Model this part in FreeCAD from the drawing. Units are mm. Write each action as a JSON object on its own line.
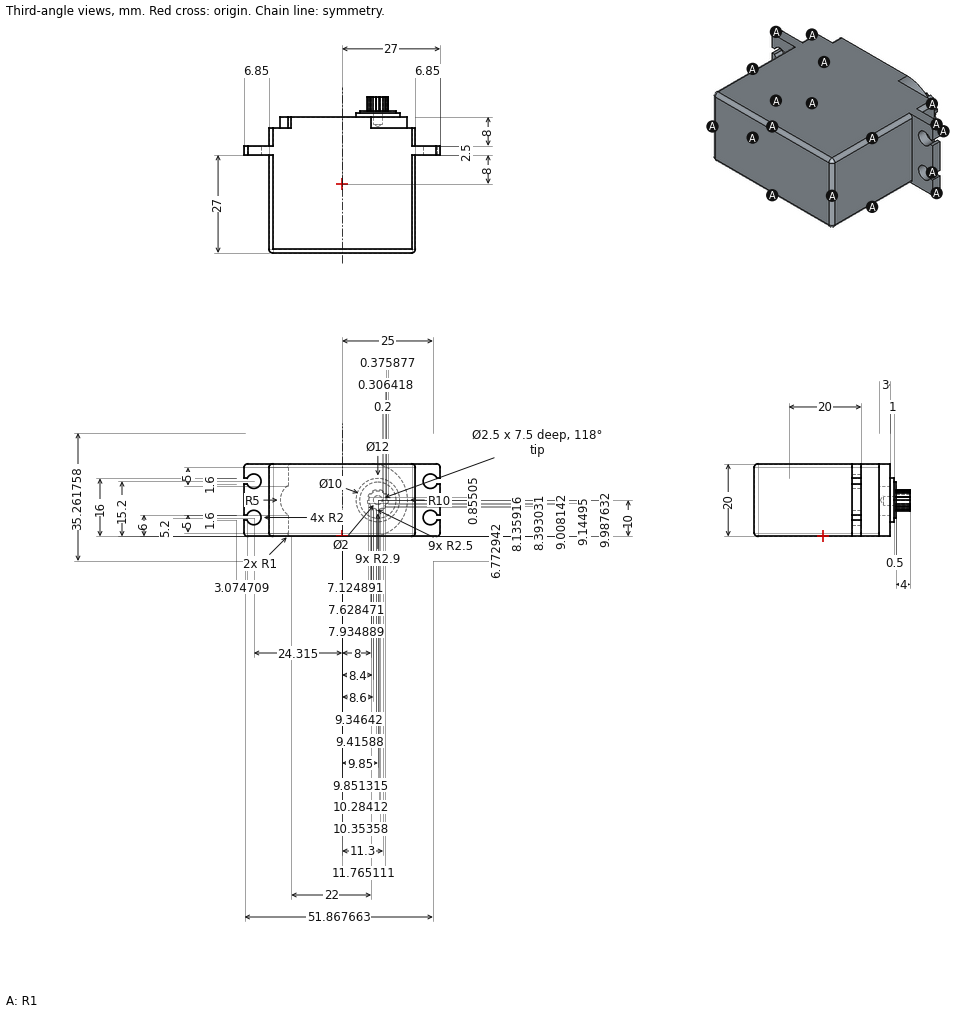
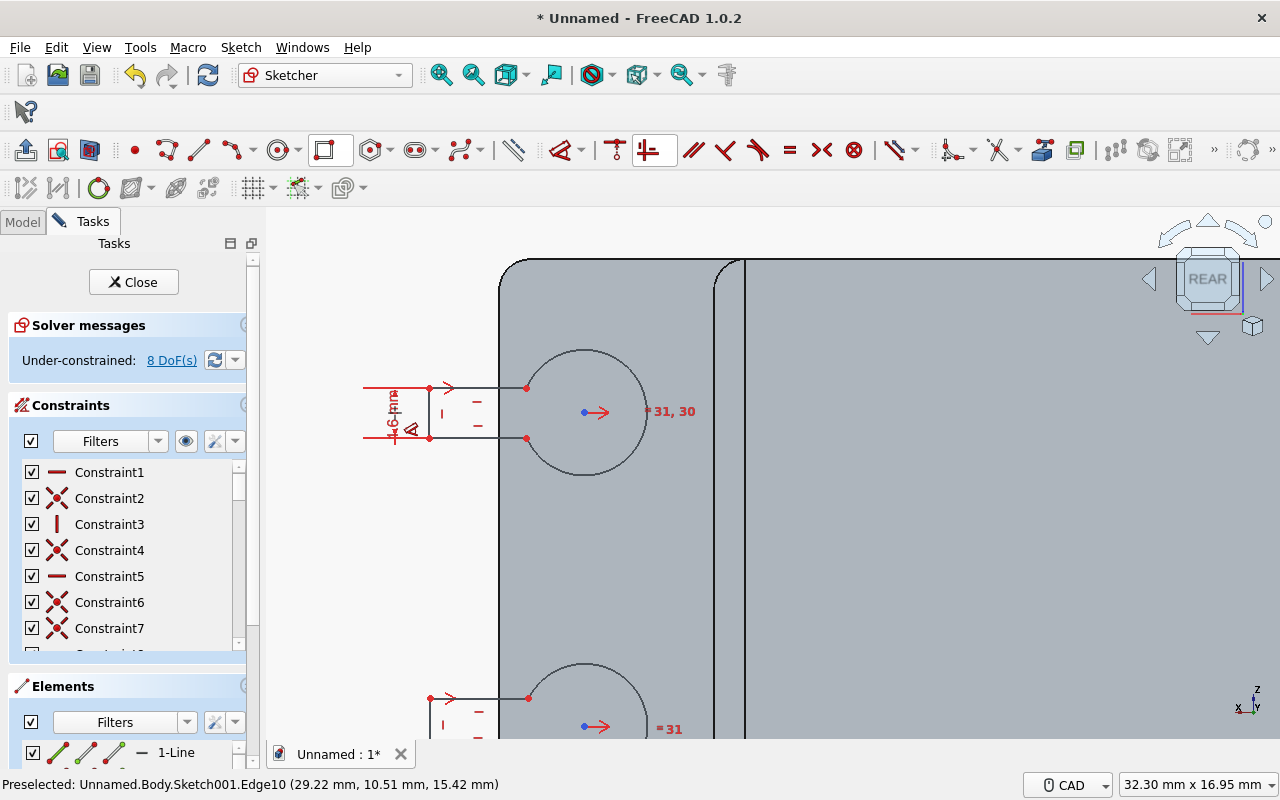
{"action": "scroll", "coordinate": [430, 709], "scroll_direction": "up", "scroll_amount": 2}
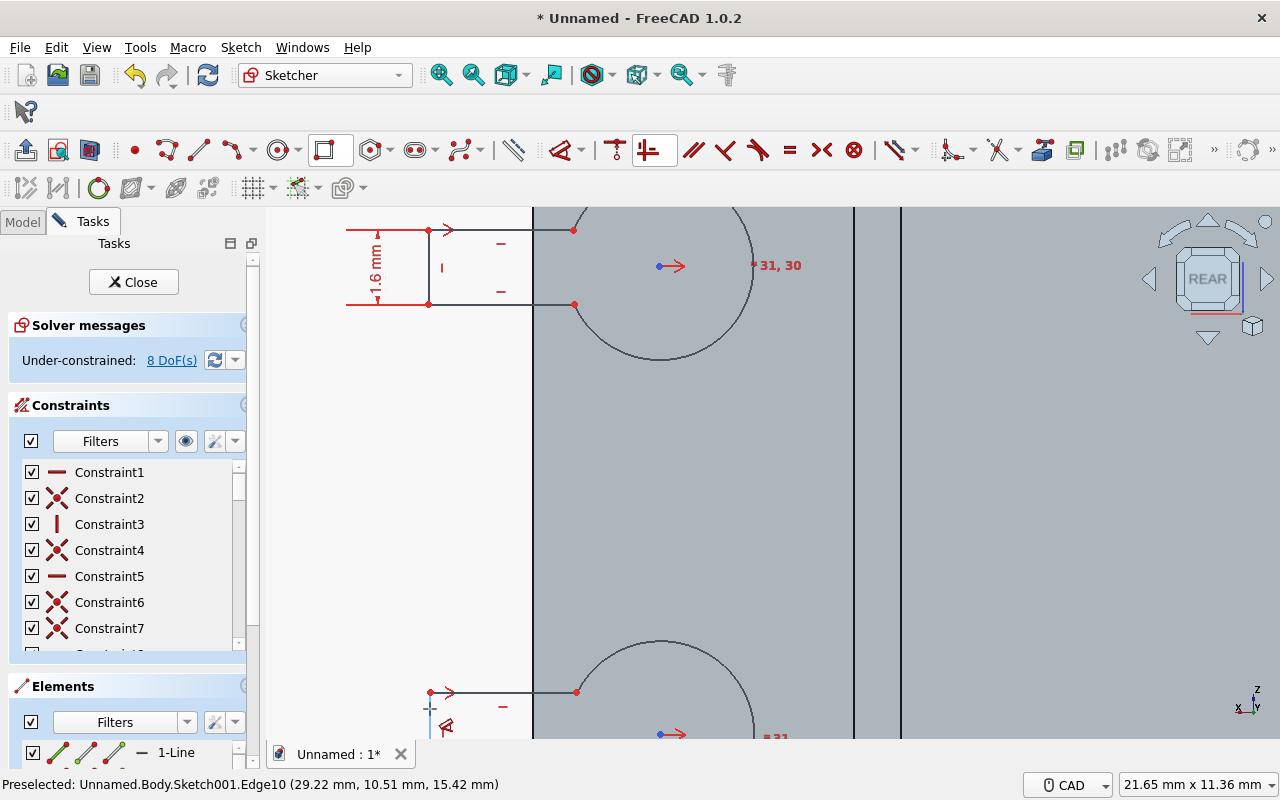
{"action": "left_click", "coordinate": [430, 709]}
{"action": "left_click", "coordinate": [396, 702]}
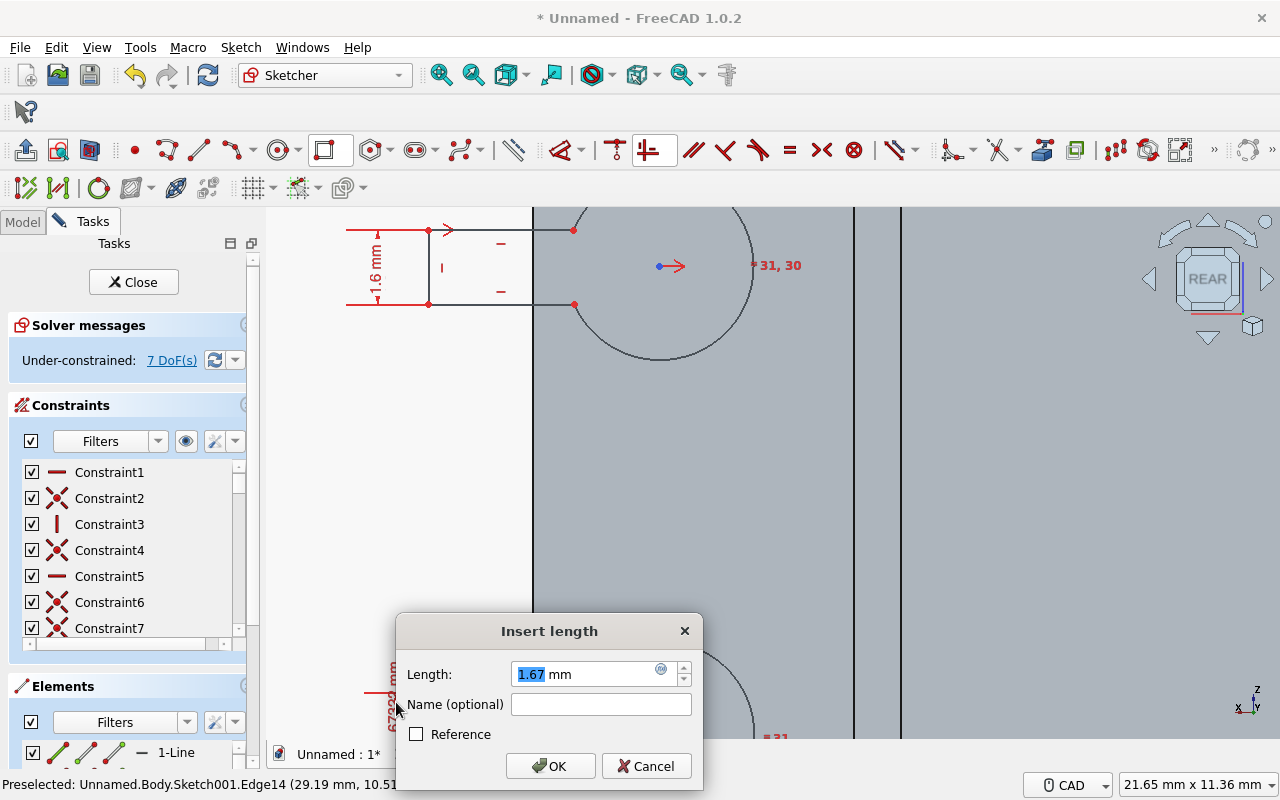
{"action": "type", "text": "1.6"}
{"action": "key", "text": "Return"}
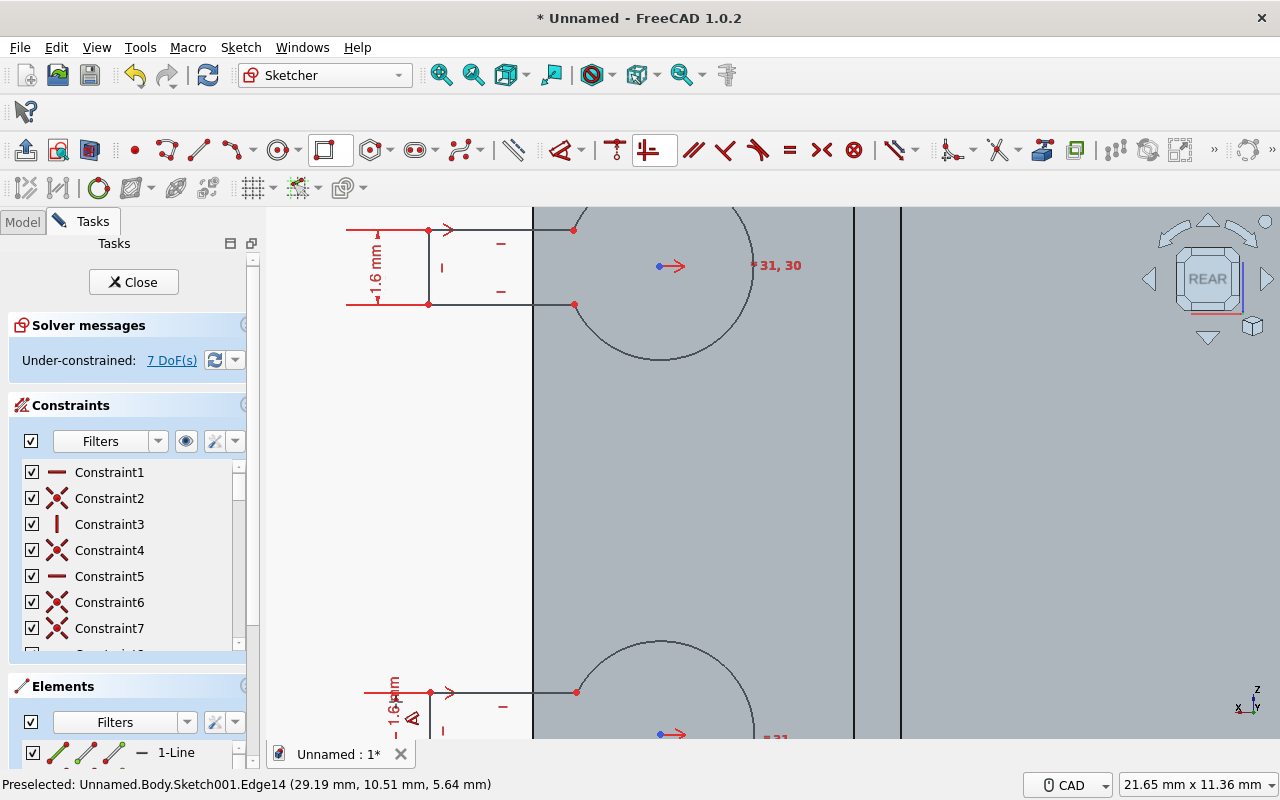
{"action": "scroll", "coordinate": [428, 441], "scroll_direction": "down", "scroll_amount": 8}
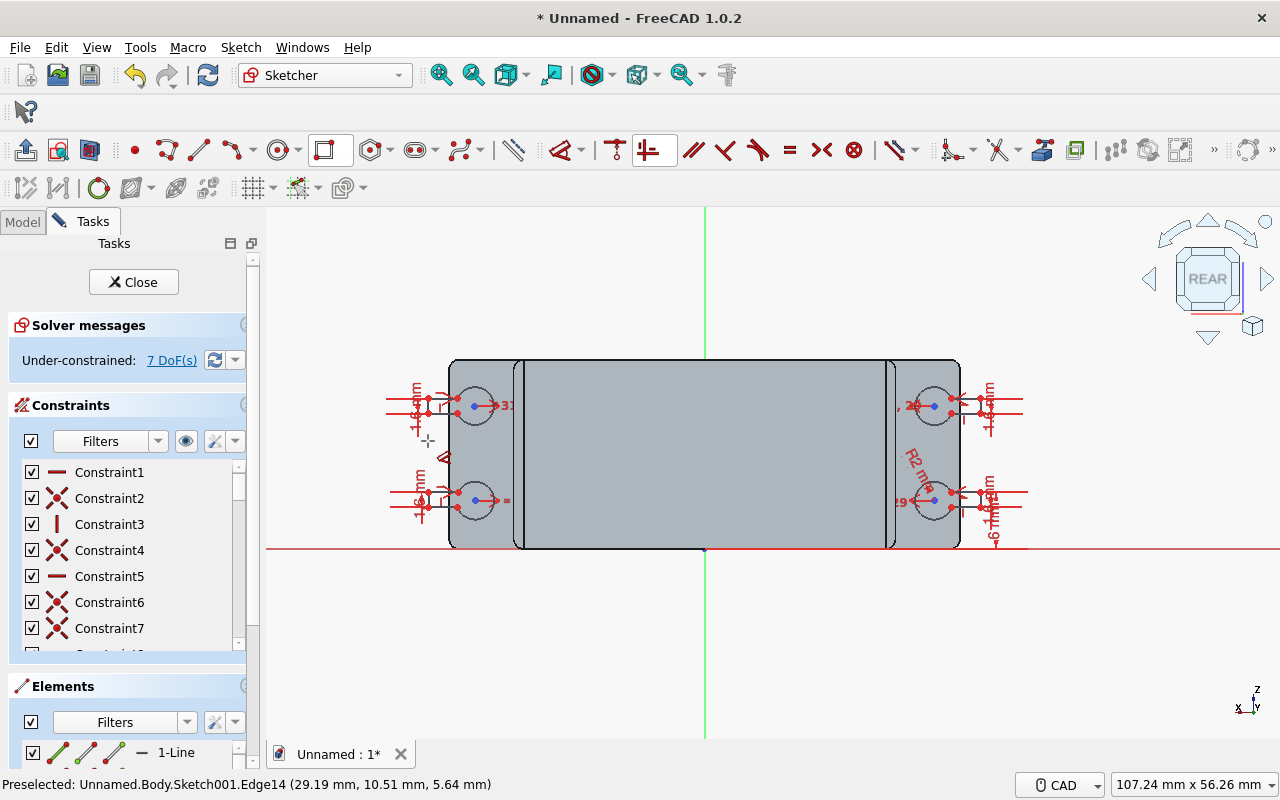
{"action": "left_click", "coordinate": [981, 399]}
{"action": "left_click", "coordinate": [1015, 474]}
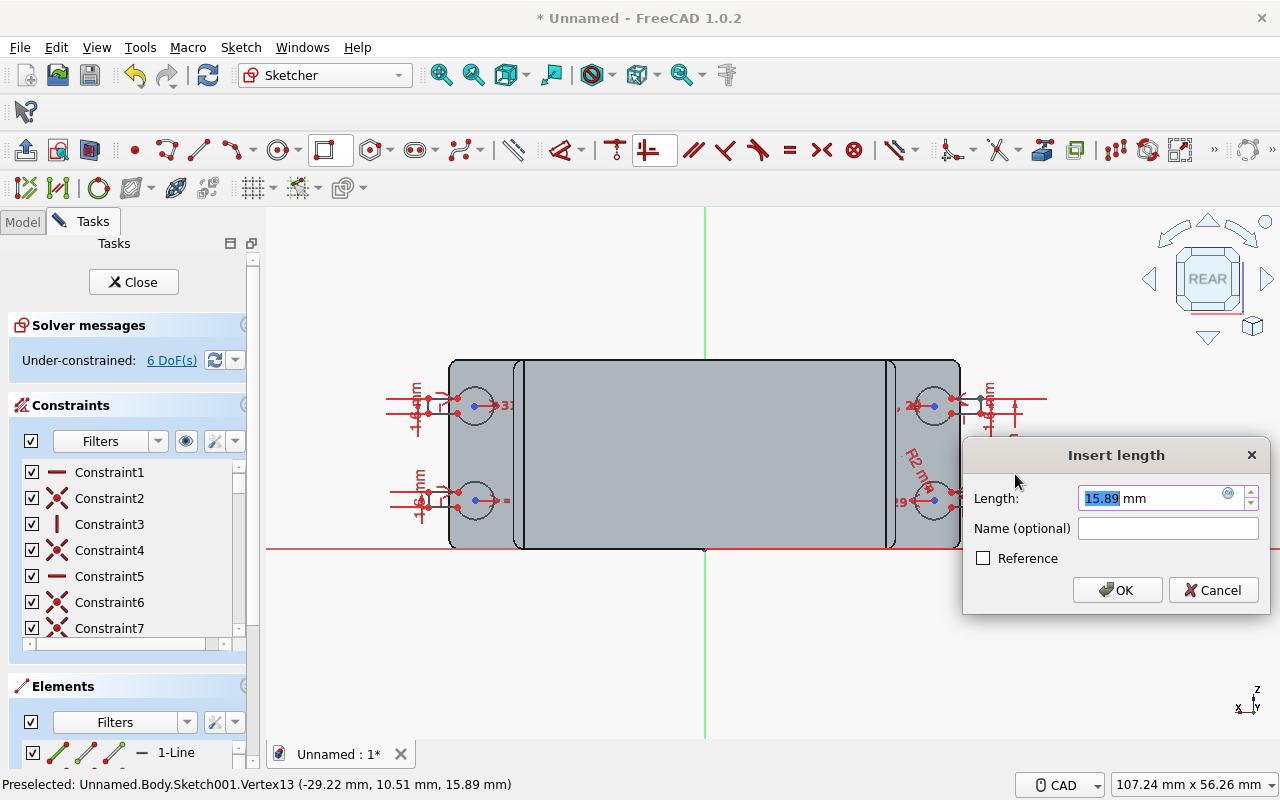
{"action": "type", "text": "16"}
{"action": "key", "text": "Return"}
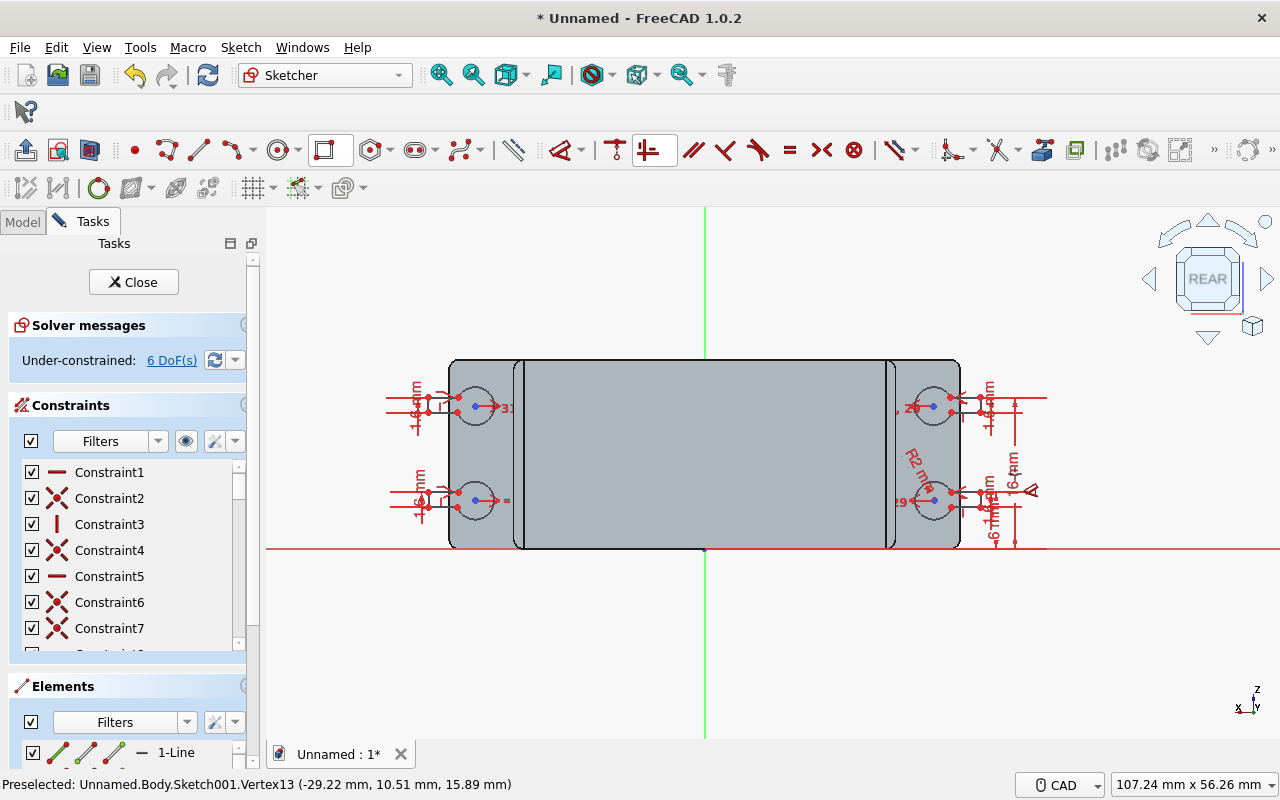
{"action": "left_click", "coordinate": [934, 501]}
{"action": "left_click", "coordinate": [671, 525]}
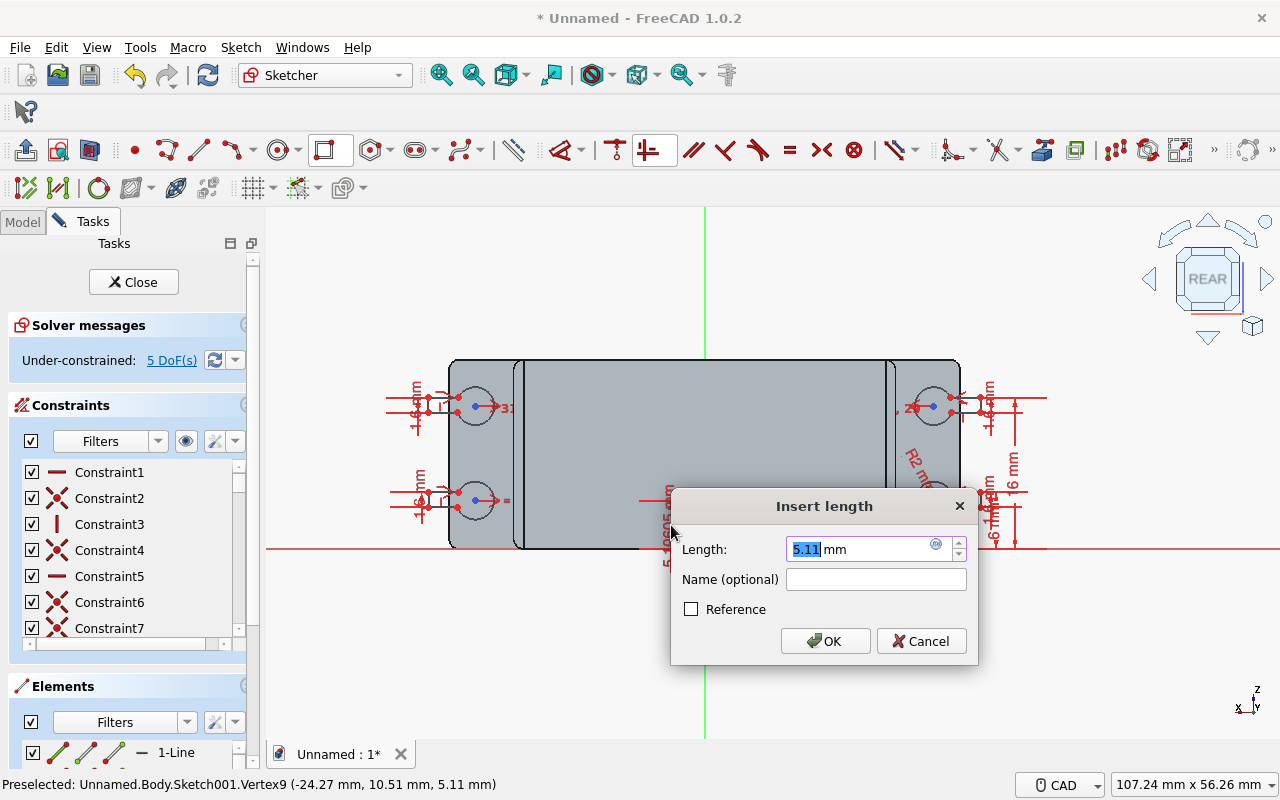
{"action": "type", "text": "5.2"}
{"action": "key", "text": "Return"}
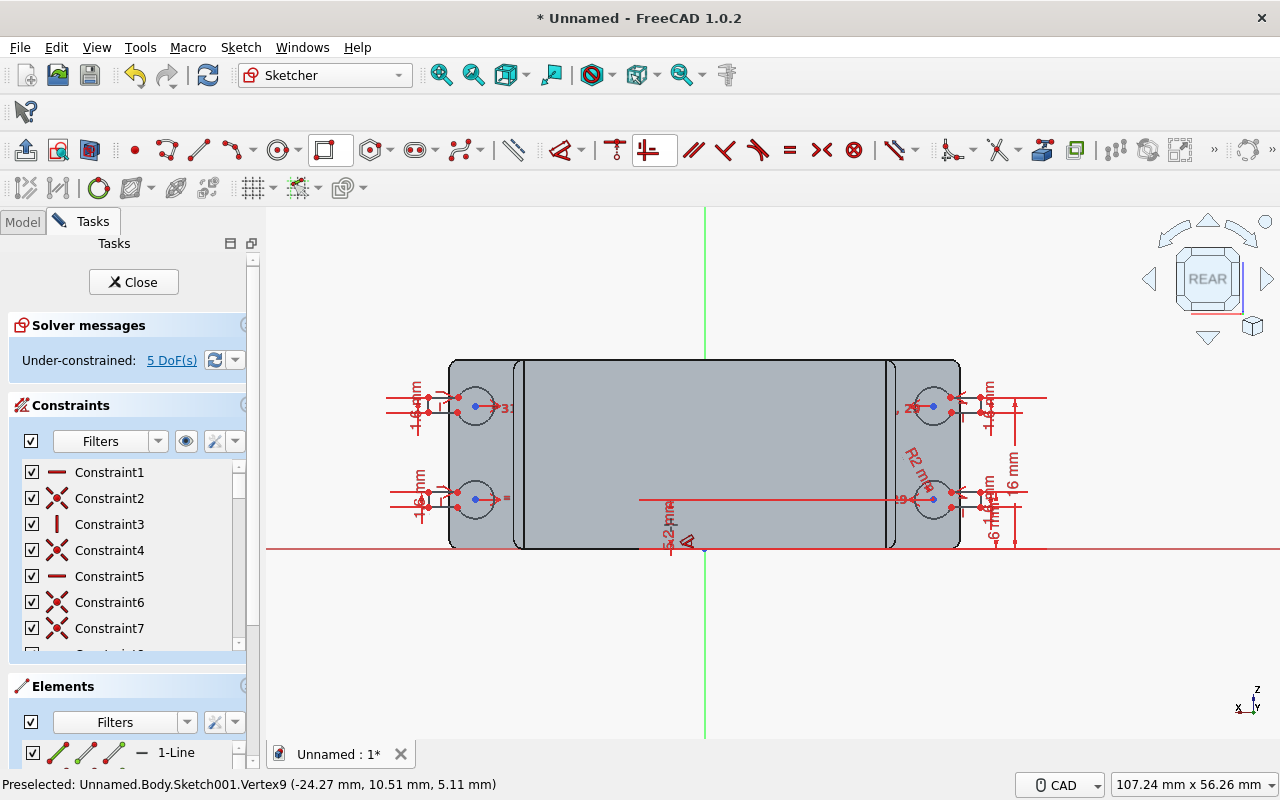
{"action": "left_click", "coordinate": [934, 406]}
{"action": "left_click", "coordinate": [968, 445]}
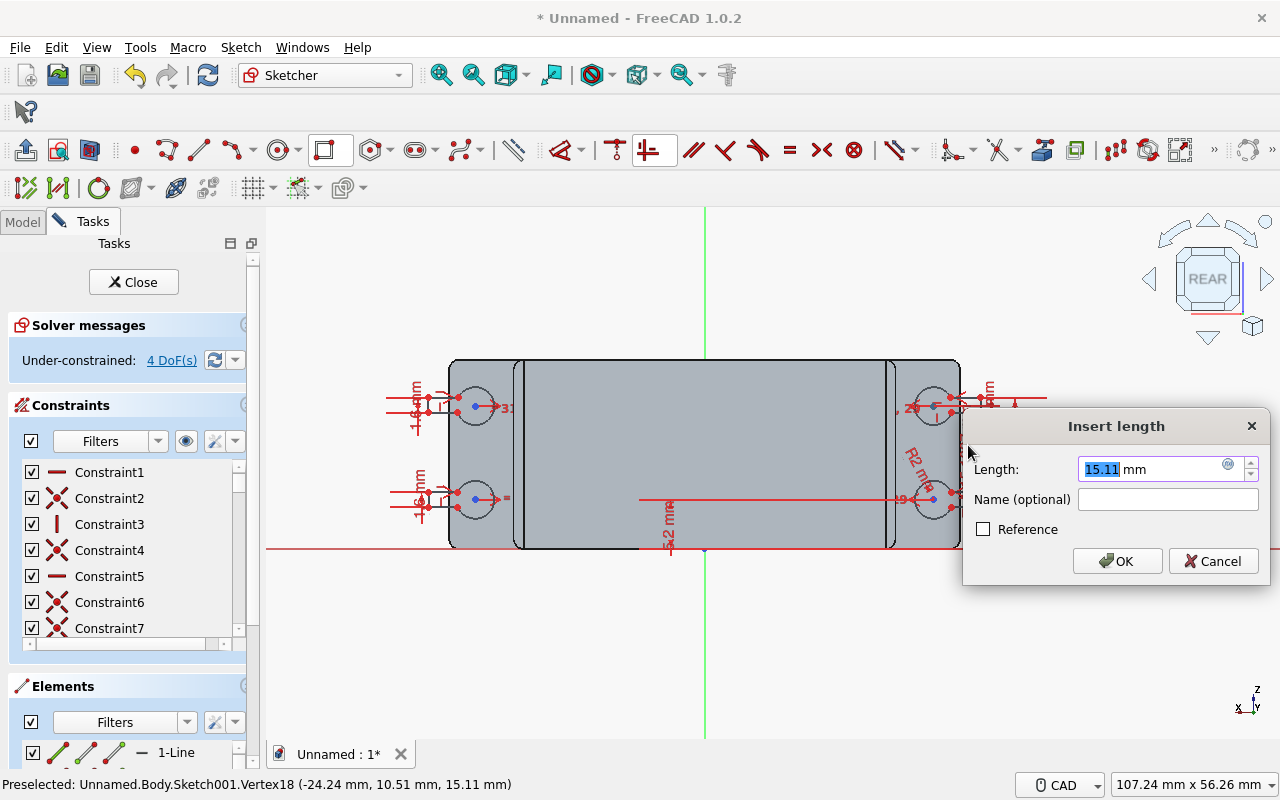
{"action": "type", "text": "15.2"}
{"action": "key", "text": "Return"}